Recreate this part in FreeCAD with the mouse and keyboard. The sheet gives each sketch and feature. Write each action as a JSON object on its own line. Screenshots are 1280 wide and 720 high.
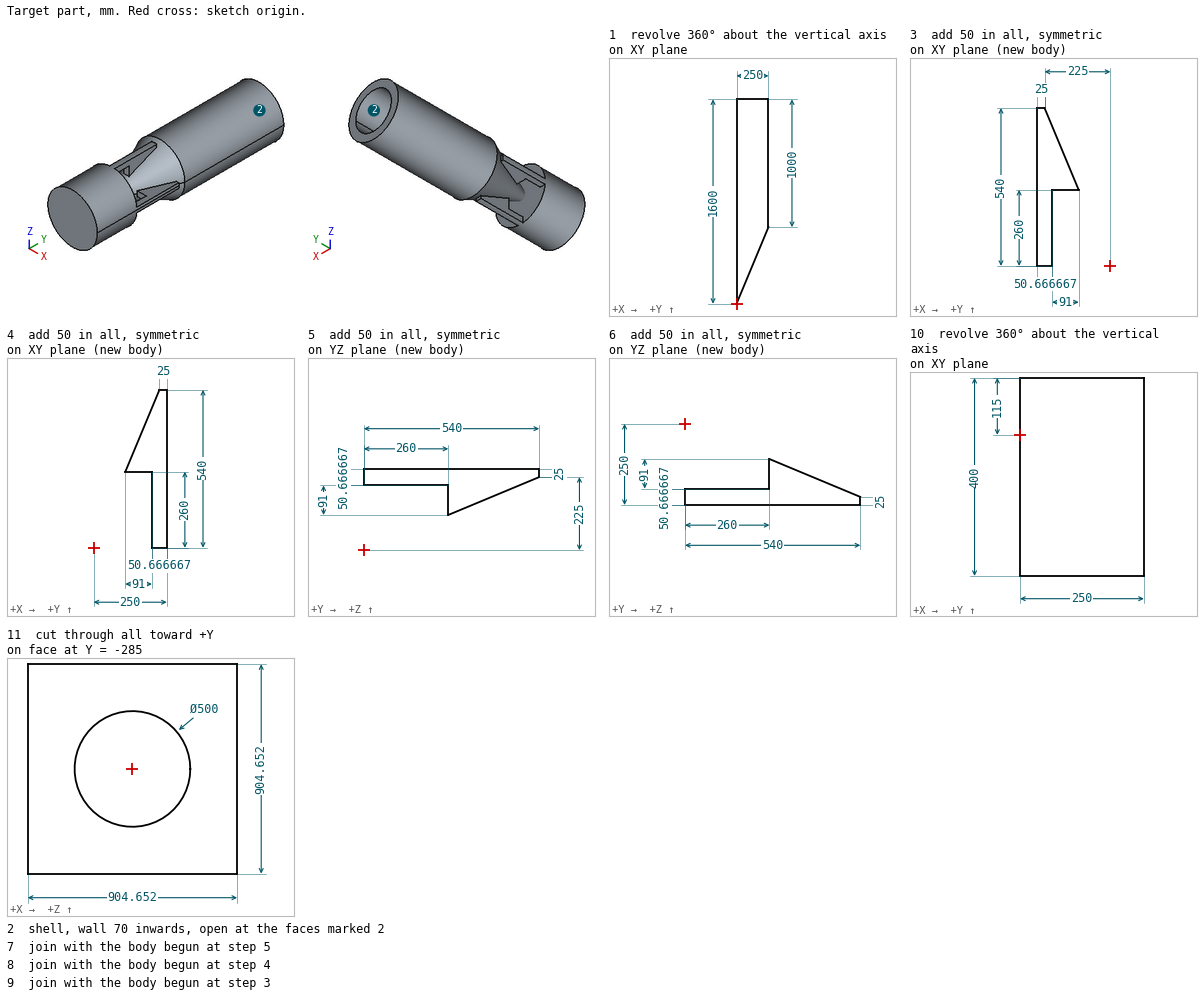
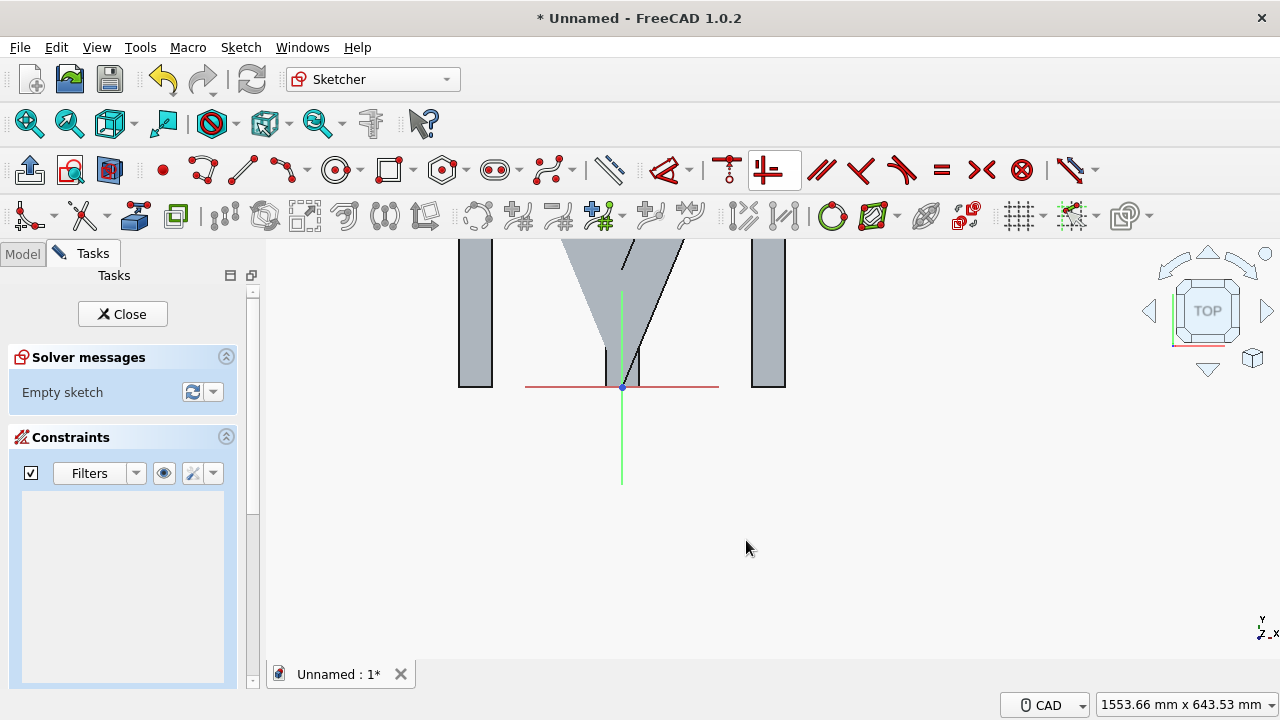
{"action": "left_click", "coordinate": [390, 170]}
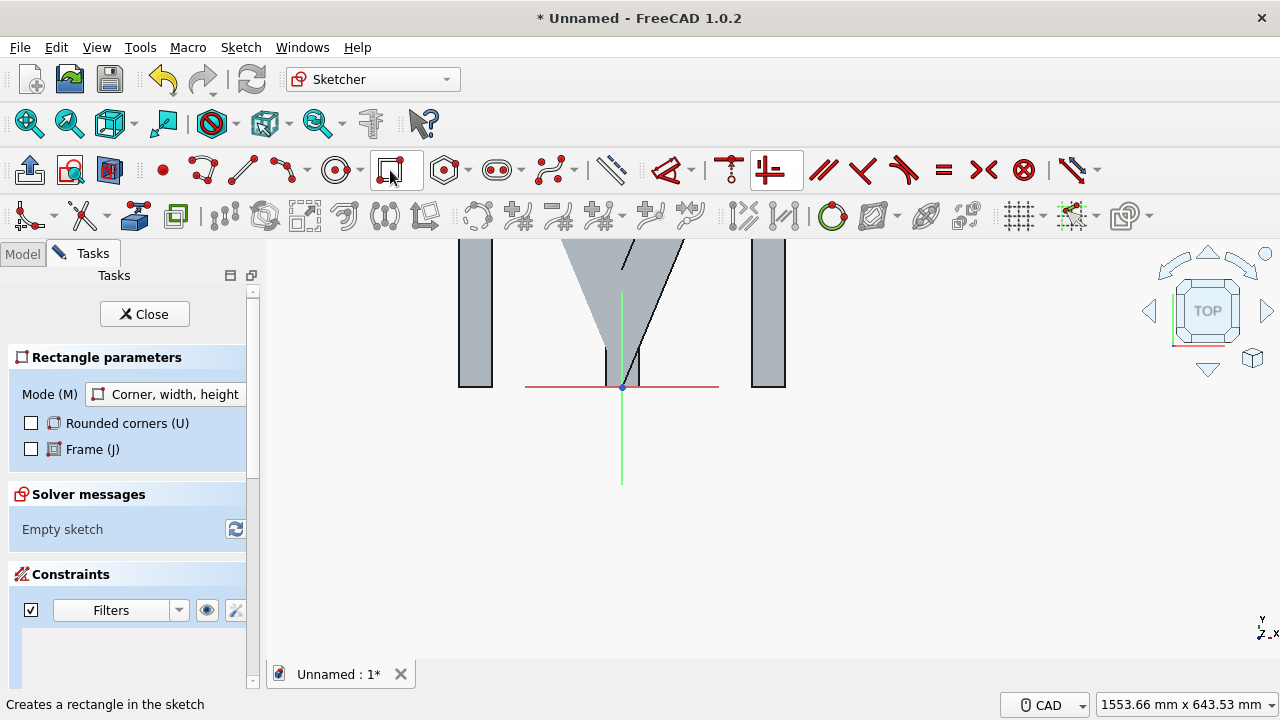
{"action": "left_click", "coordinate": [622, 312]}
{"action": "left_click", "coordinate": [785, 573]}
{"action": "key", "text": "Escape"}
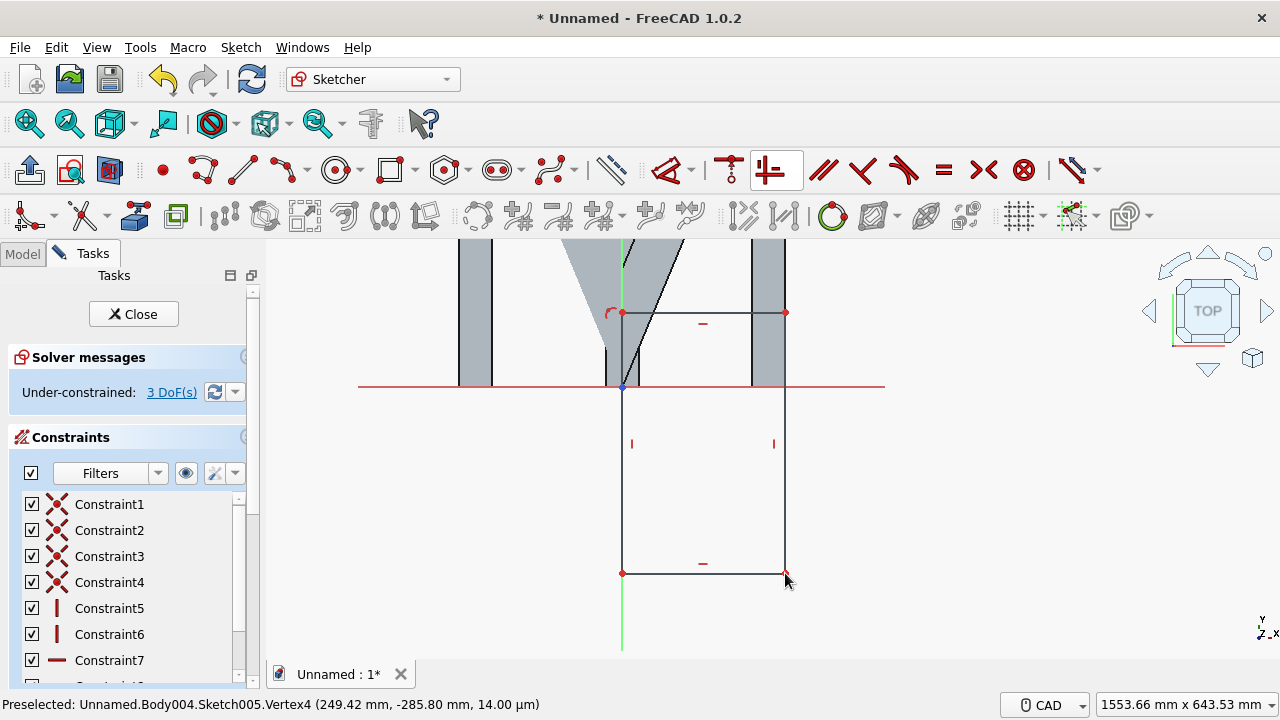
{"action": "left_click", "coordinate": [666, 170]}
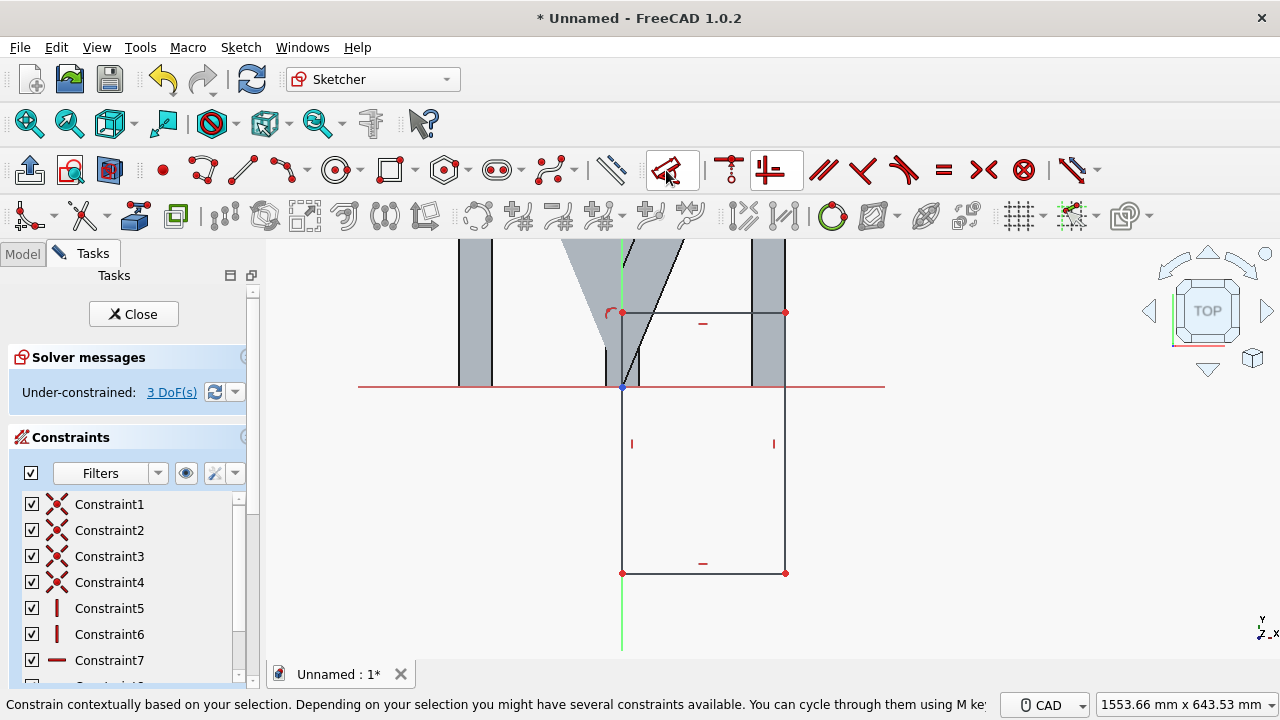
{"action": "left_click", "coordinate": [622, 496]}
{"action": "left_click", "coordinate": [588, 444]}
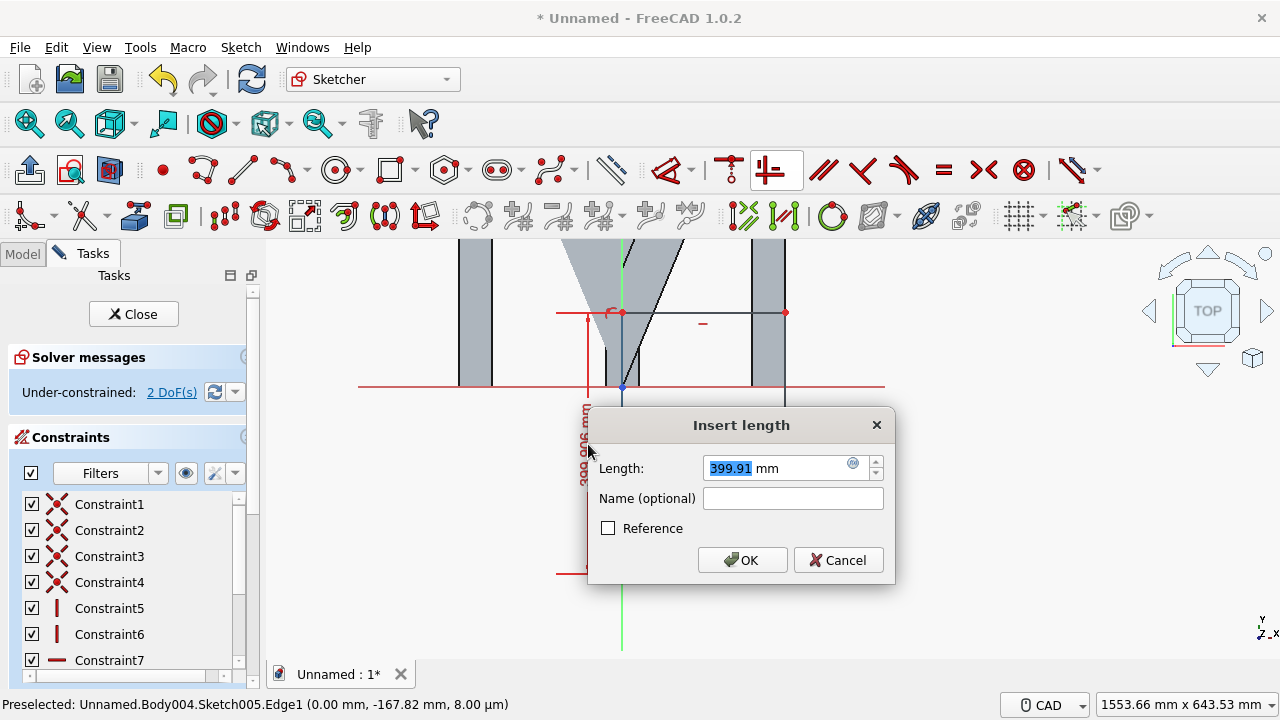
{"action": "type", "text": "400"}
{"action": "key", "text": "Return"}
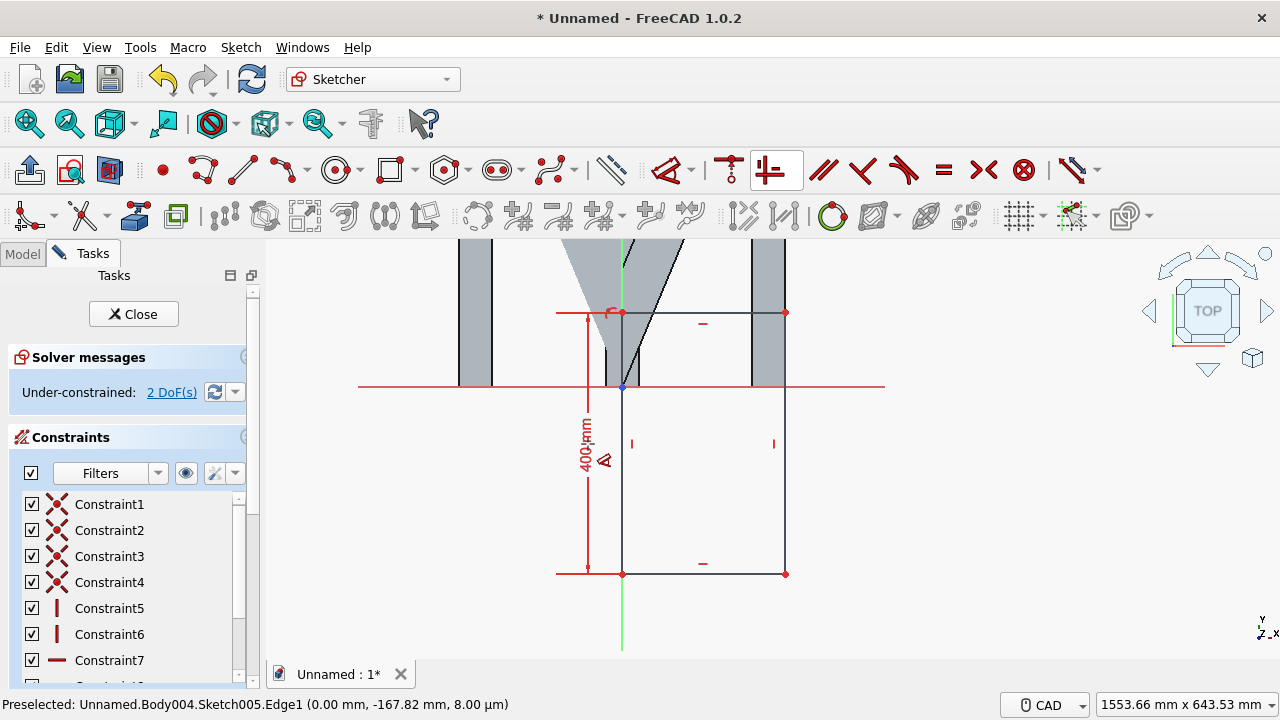
{"action": "left_click", "coordinate": [671, 574]}
{"action": "left_click", "coordinate": [704, 608]}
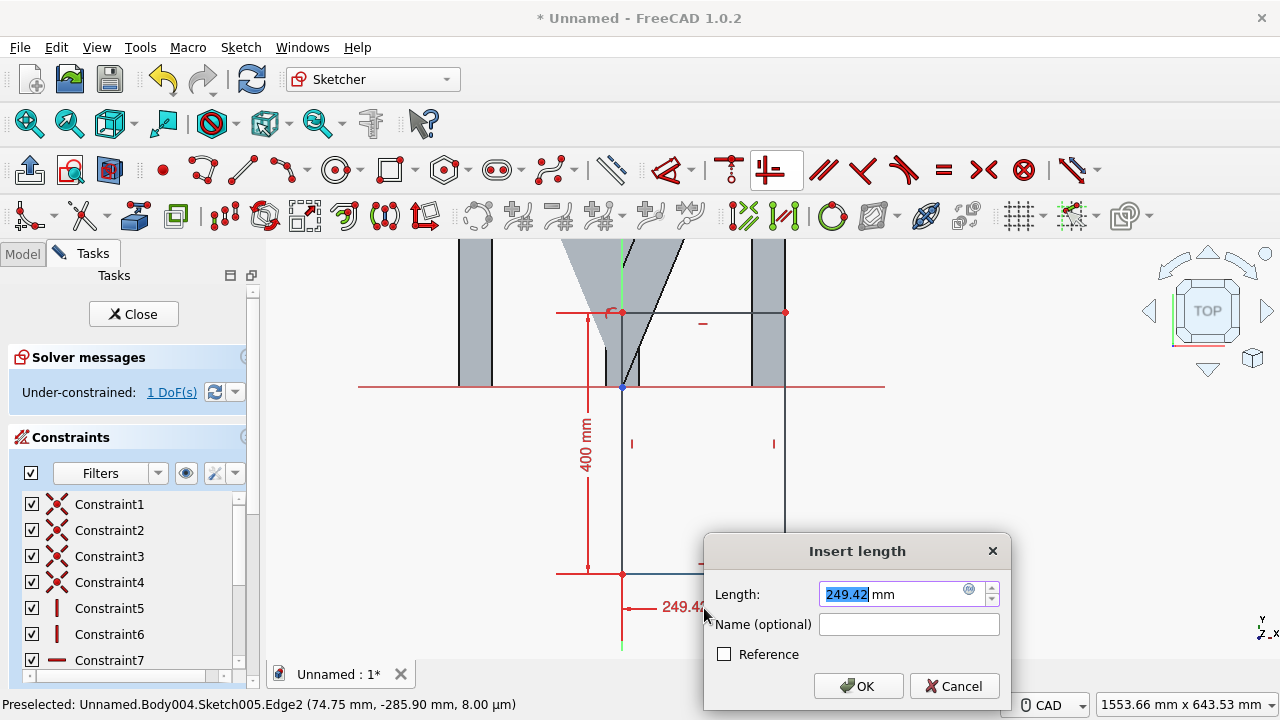
{"action": "type", "text": "250"}
{"action": "key", "text": "Return"}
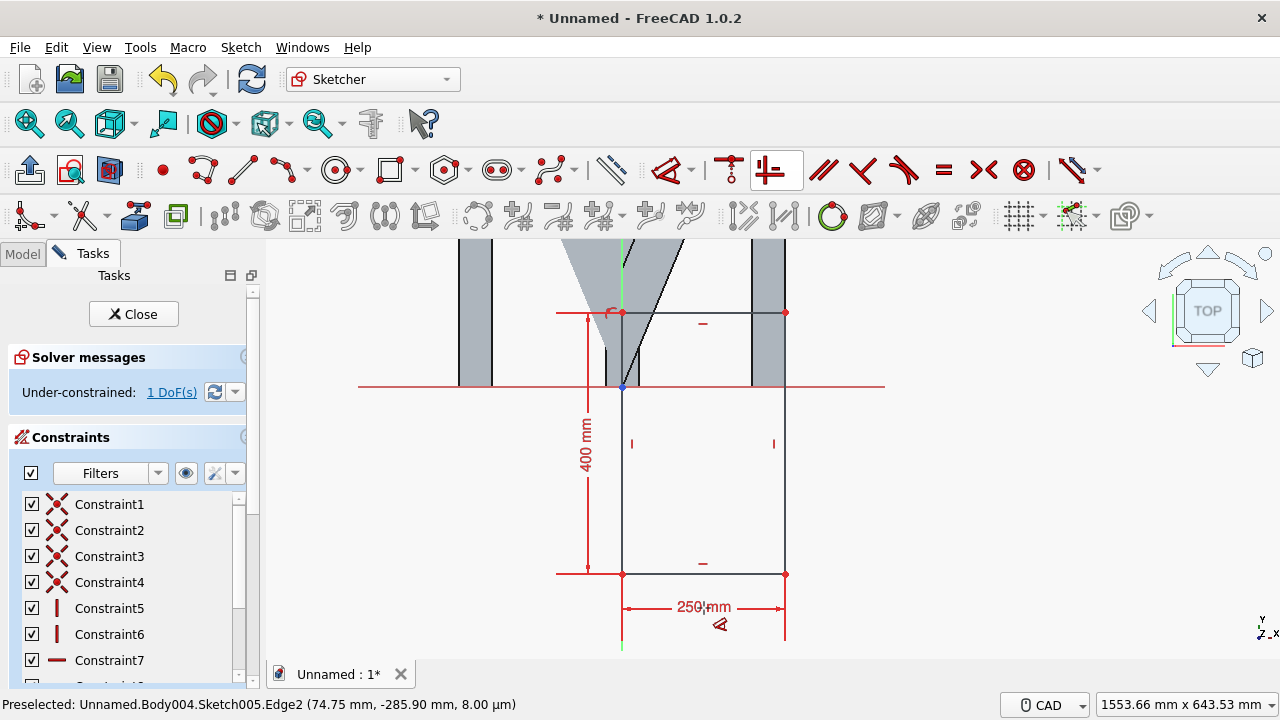
{"action": "left_click", "coordinate": [622, 313]}
{"action": "left_click", "coordinate": [588, 350]}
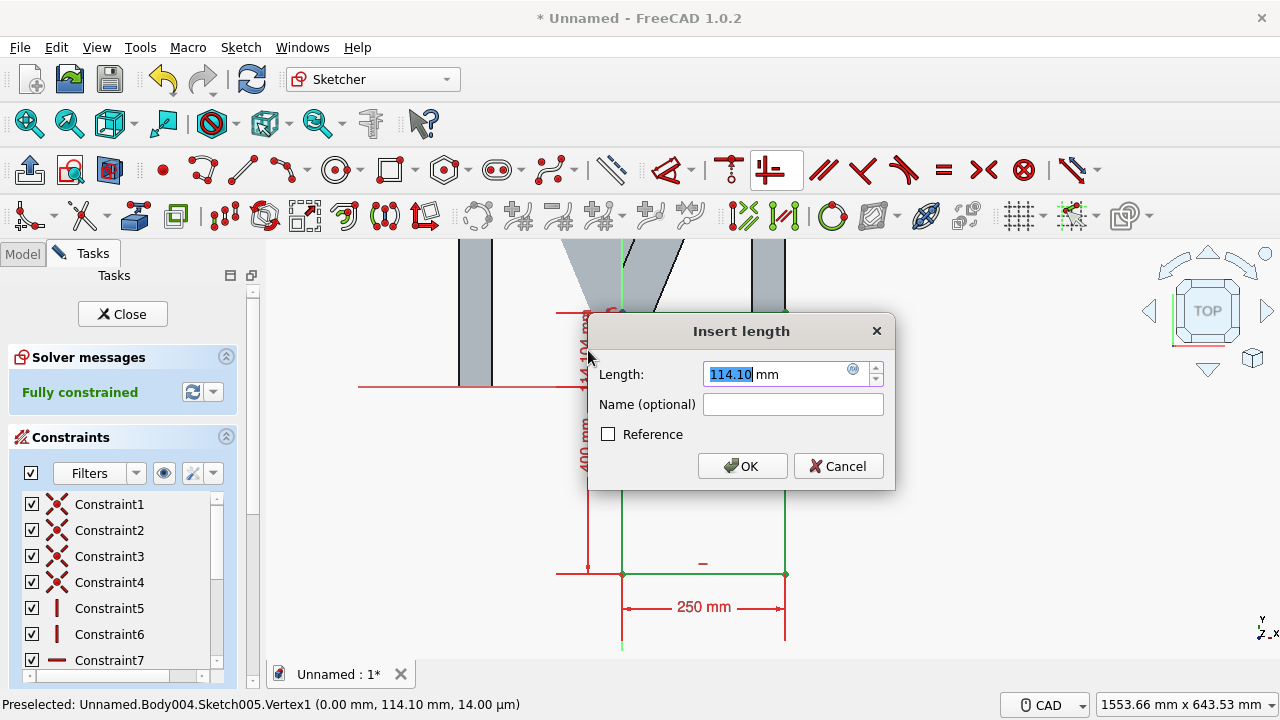
{"action": "type", "text": "115"}
{"action": "key", "text": "Return"}
{"action": "key", "text": "Escape"}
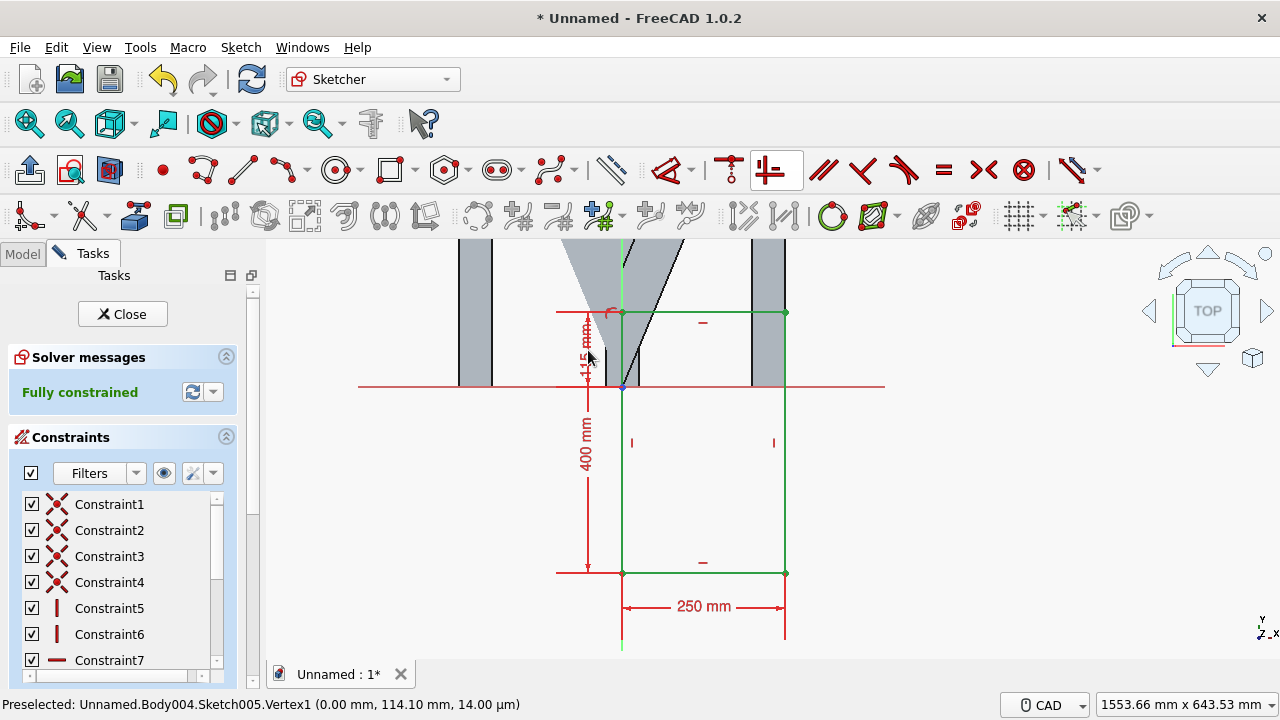
{"action": "left_click", "coordinate": [123, 314]}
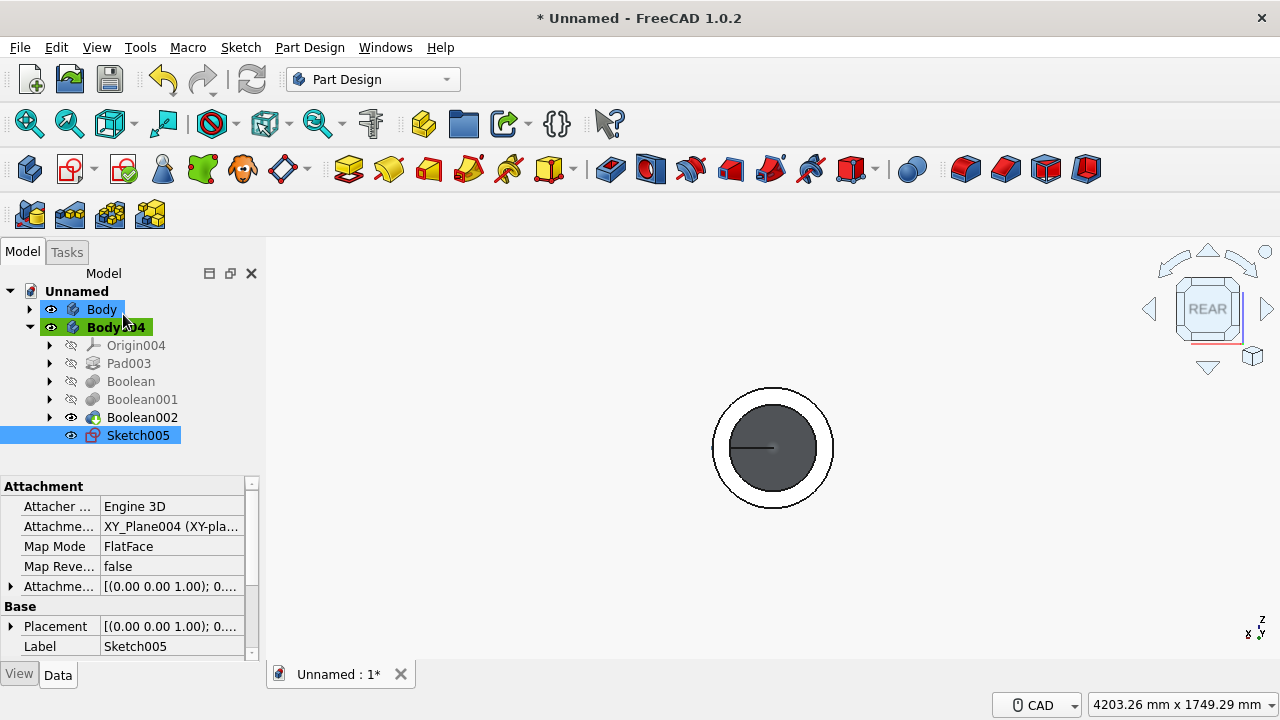
{"action": "left_click", "coordinate": [390, 170]}